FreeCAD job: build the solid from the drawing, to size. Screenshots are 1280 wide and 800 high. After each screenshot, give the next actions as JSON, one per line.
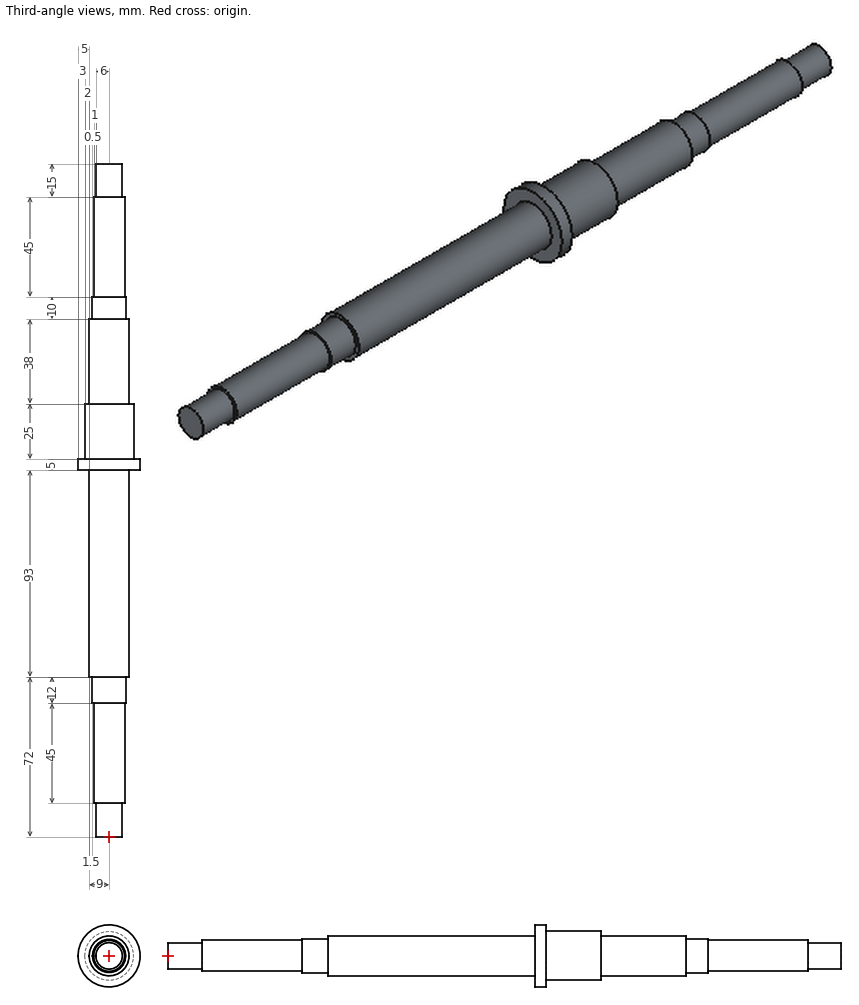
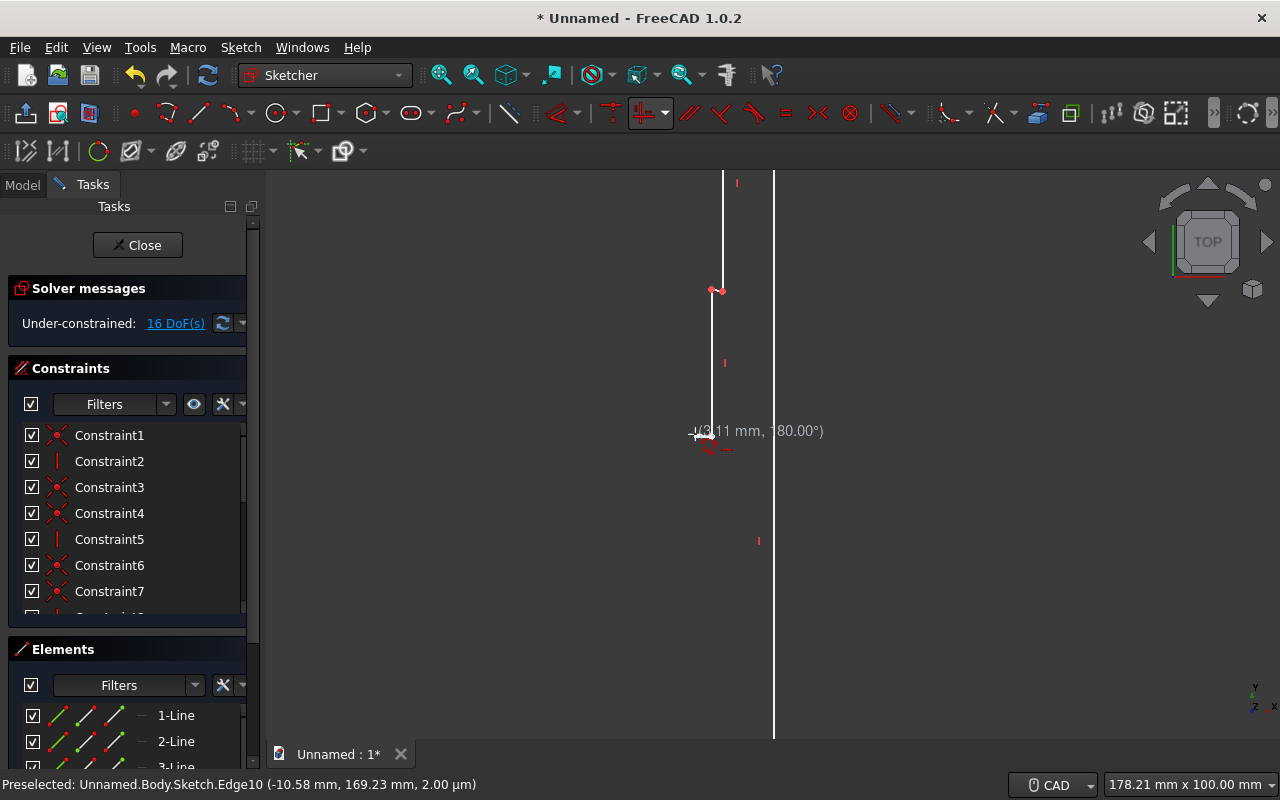
{"action": "left_click", "coordinate": [694, 433]}
{"action": "left_click", "coordinate": [694, 460]}
{"action": "left_click", "coordinate": [723, 460]}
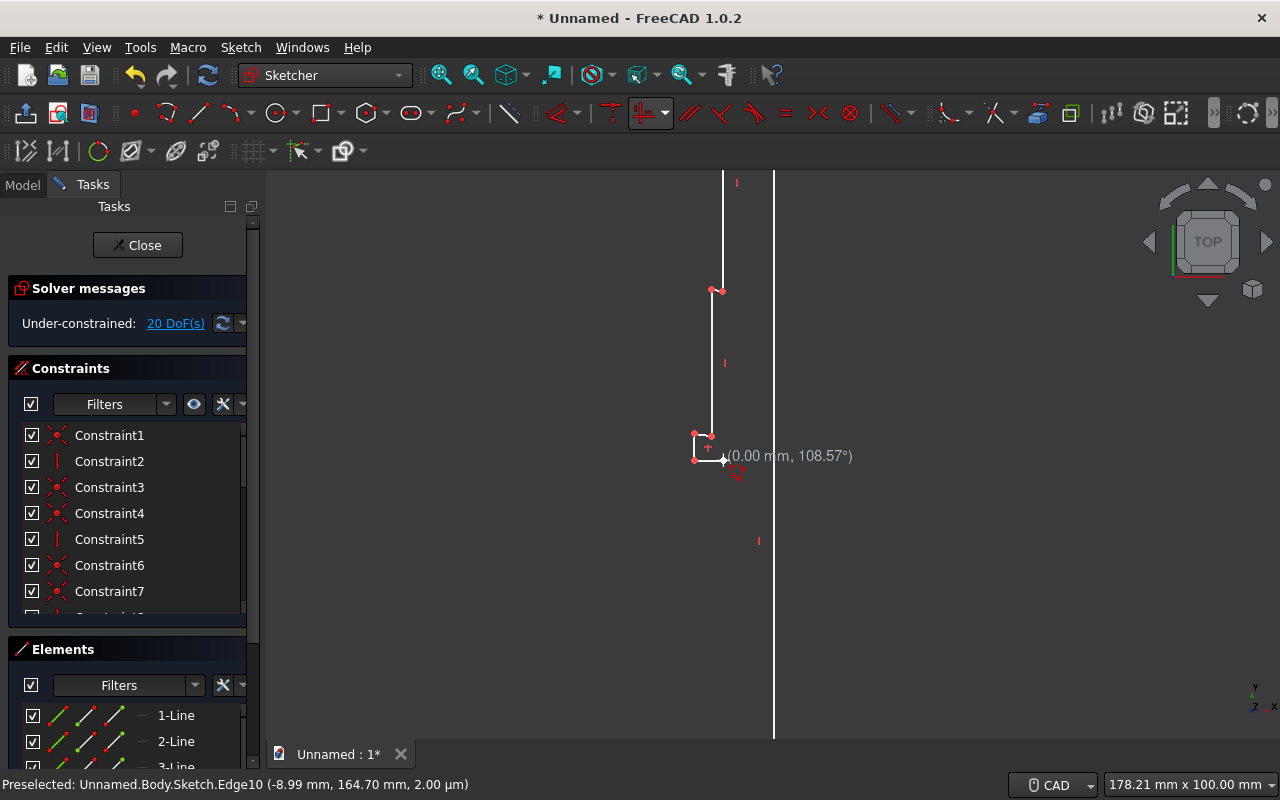
{"action": "scroll", "coordinate": [697, 434], "scroll_direction": "down", "scroll_amount": 8}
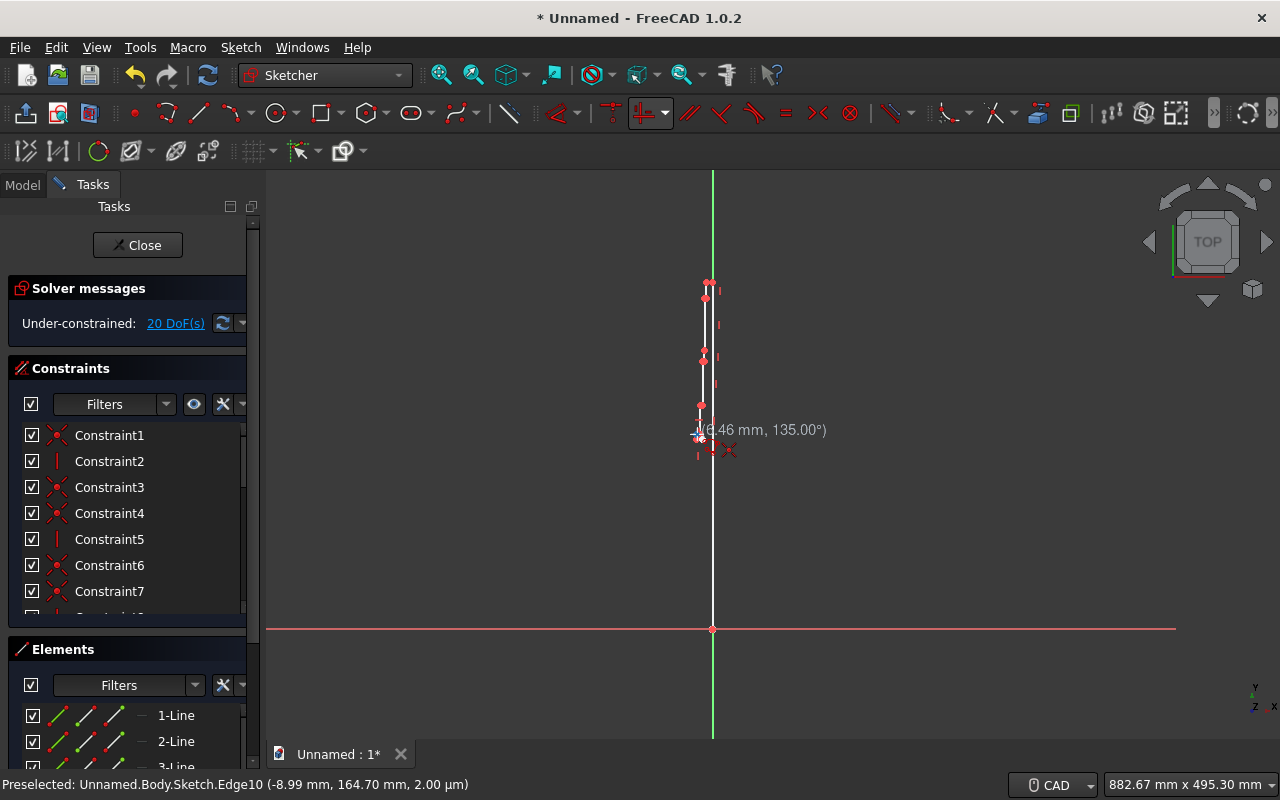
{"action": "scroll", "coordinate": [703, 547], "scroll_direction": "up", "scroll_amount": 3}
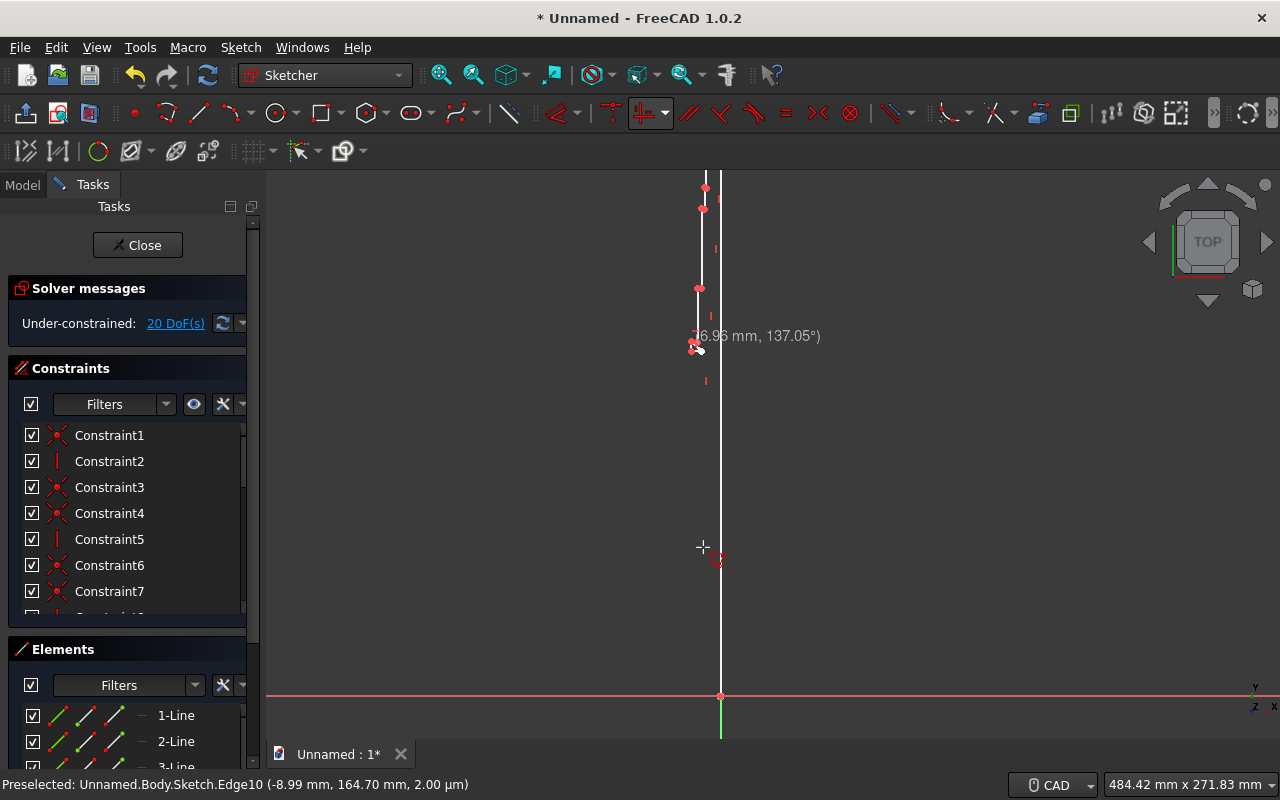
{"action": "left_click", "coordinate": [702, 546]}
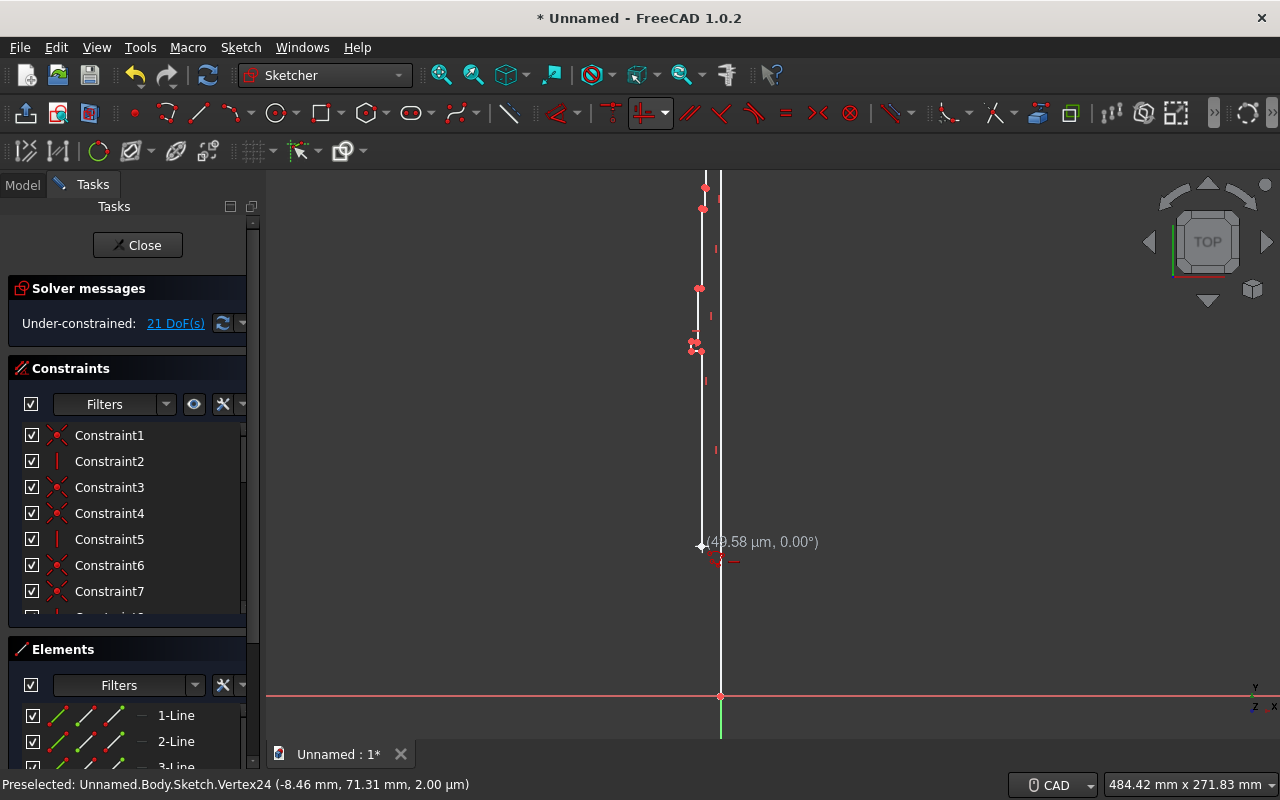
{"action": "scroll", "coordinate": [705, 546], "scroll_direction": "up", "scroll_amount": 9}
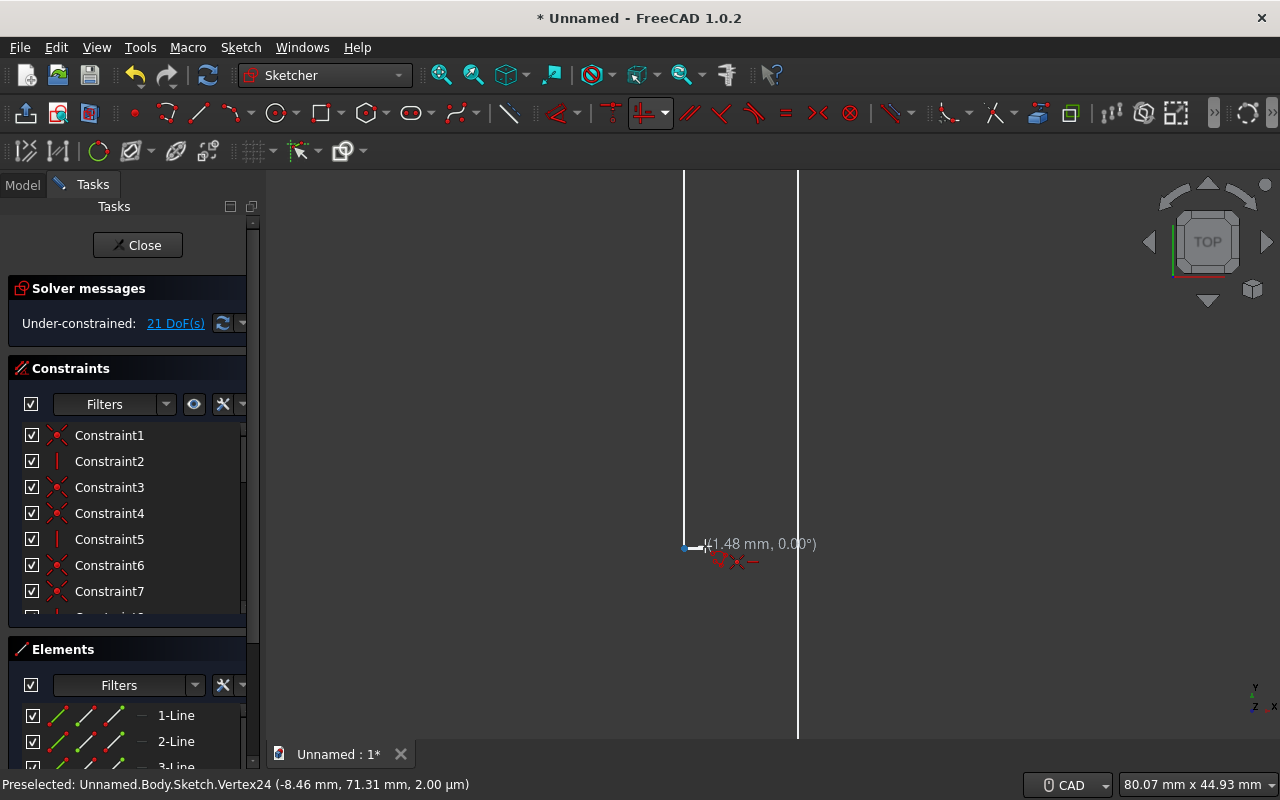
{"action": "left_click", "coordinate": [703, 543]}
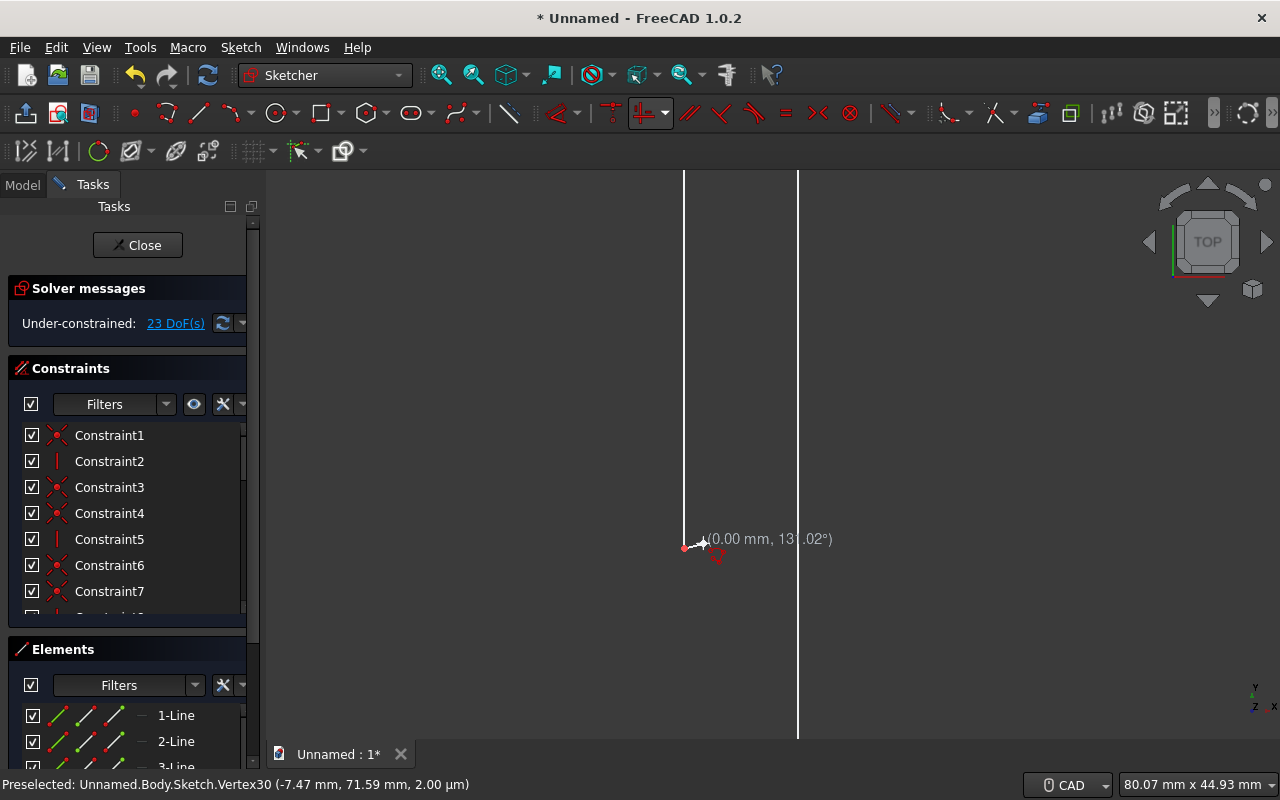
{"action": "scroll", "coordinate": [704, 546], "scroll_direction": "down", "scroll_amount": 12}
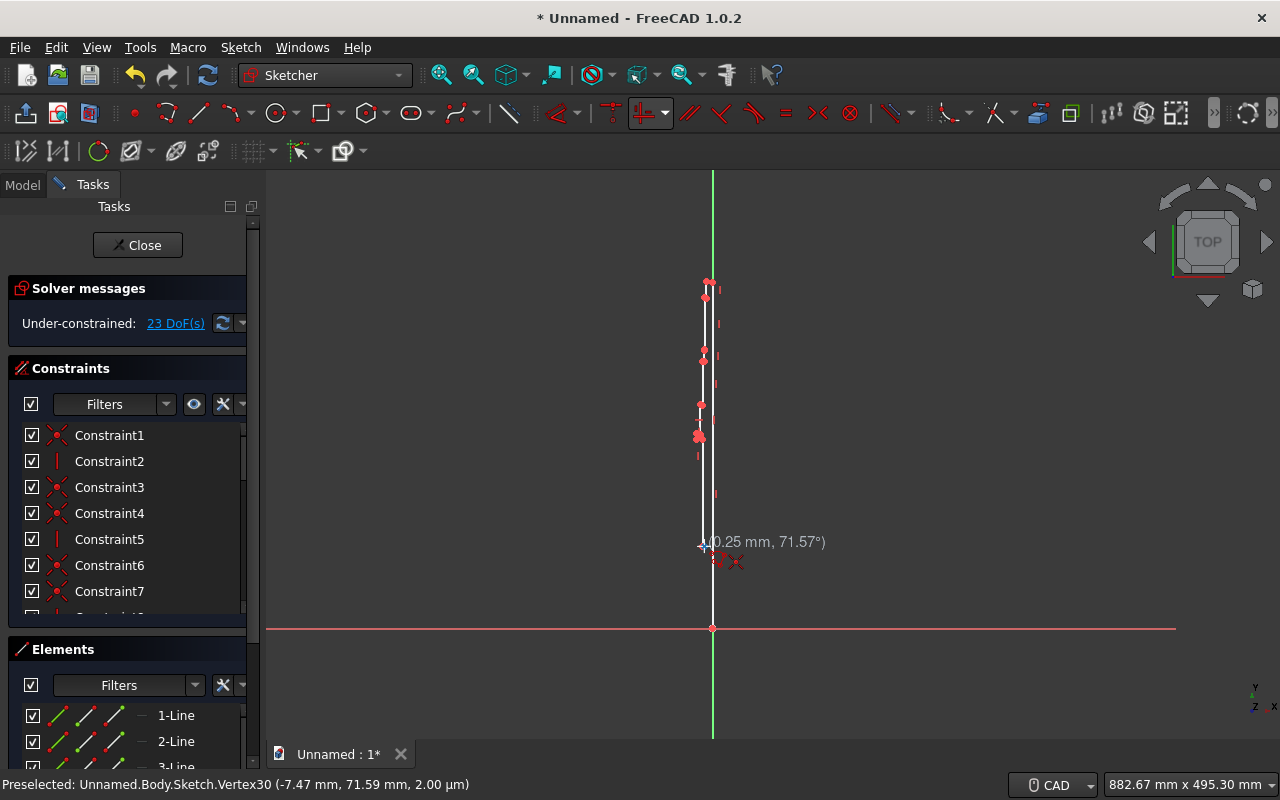
{"action": "scroll", "coordinate": [704, 560], "scroll_direction": "up", "scroll_amount": 4}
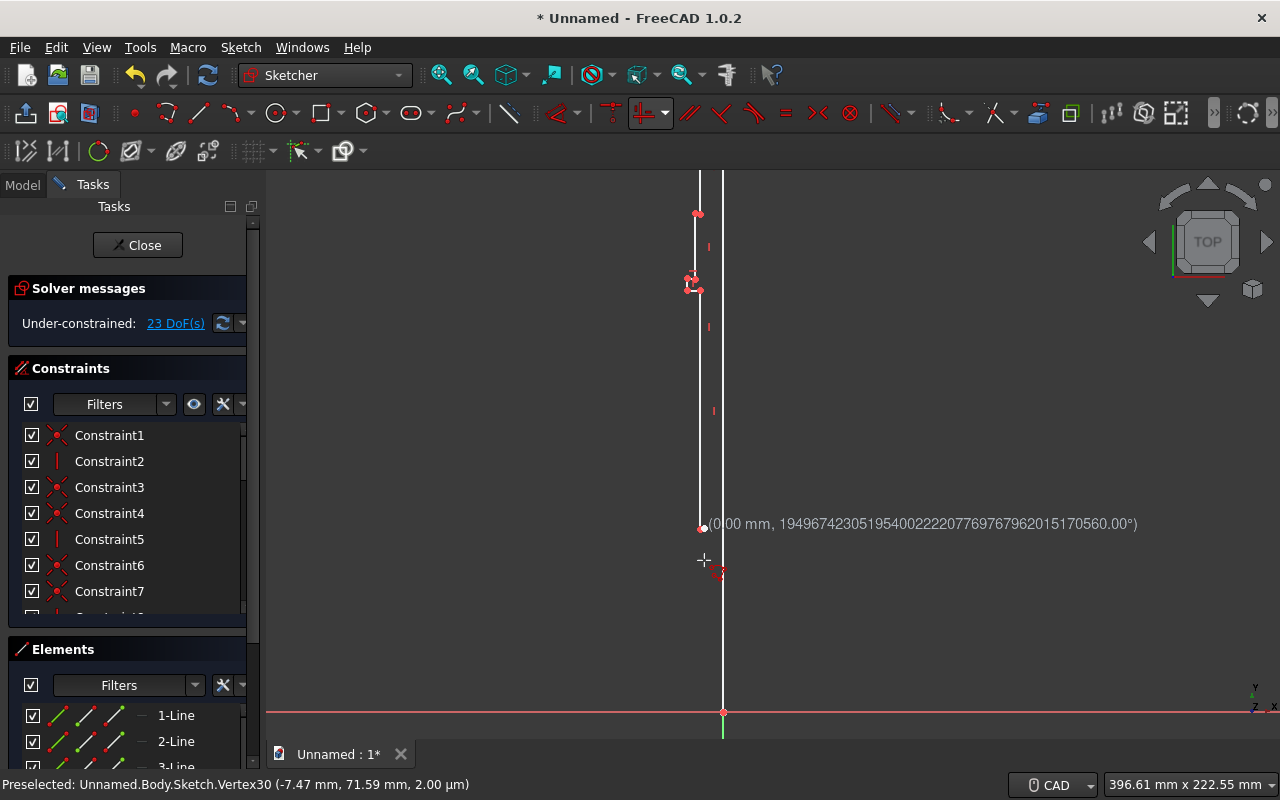
{"action": "left_click", "coordinate": [704, 559]}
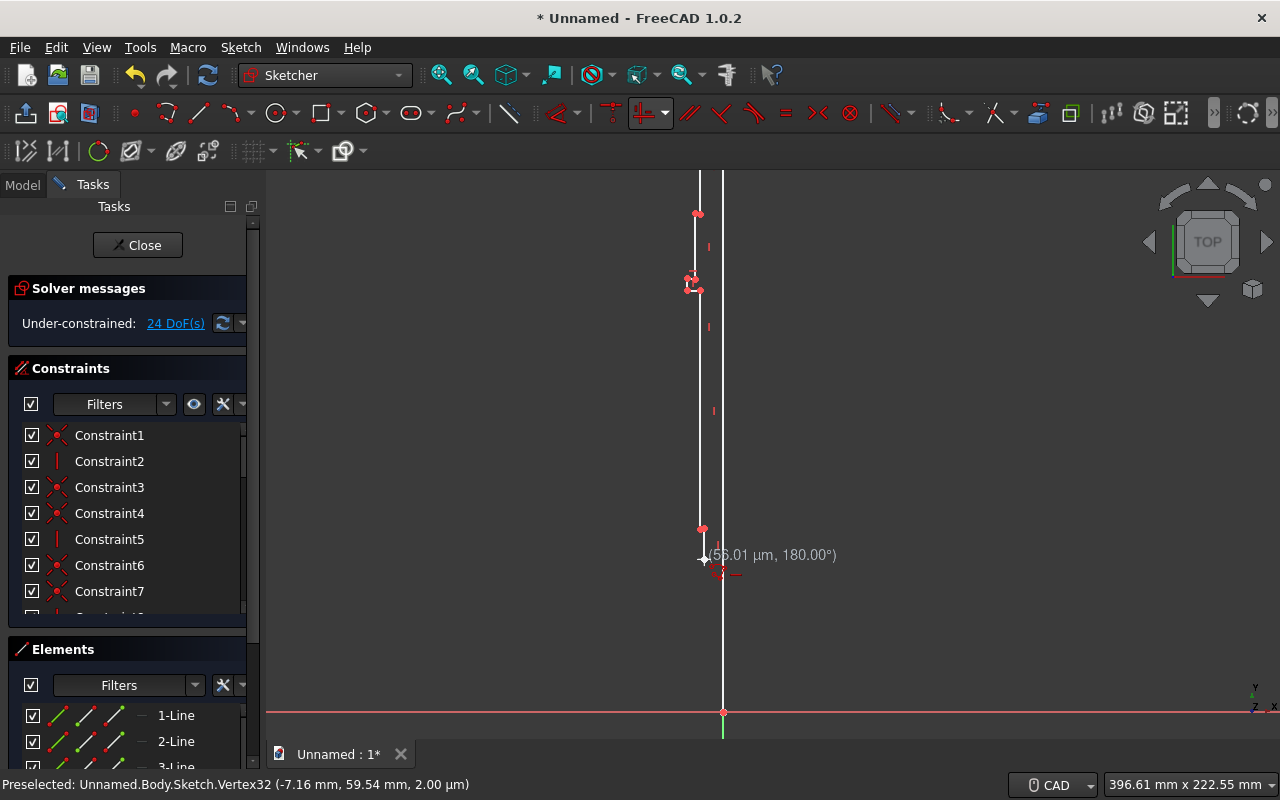
{"action": "scroll", "coordinate": [705, 559], "scroll_direction": "up", "scroll_amount": 13}